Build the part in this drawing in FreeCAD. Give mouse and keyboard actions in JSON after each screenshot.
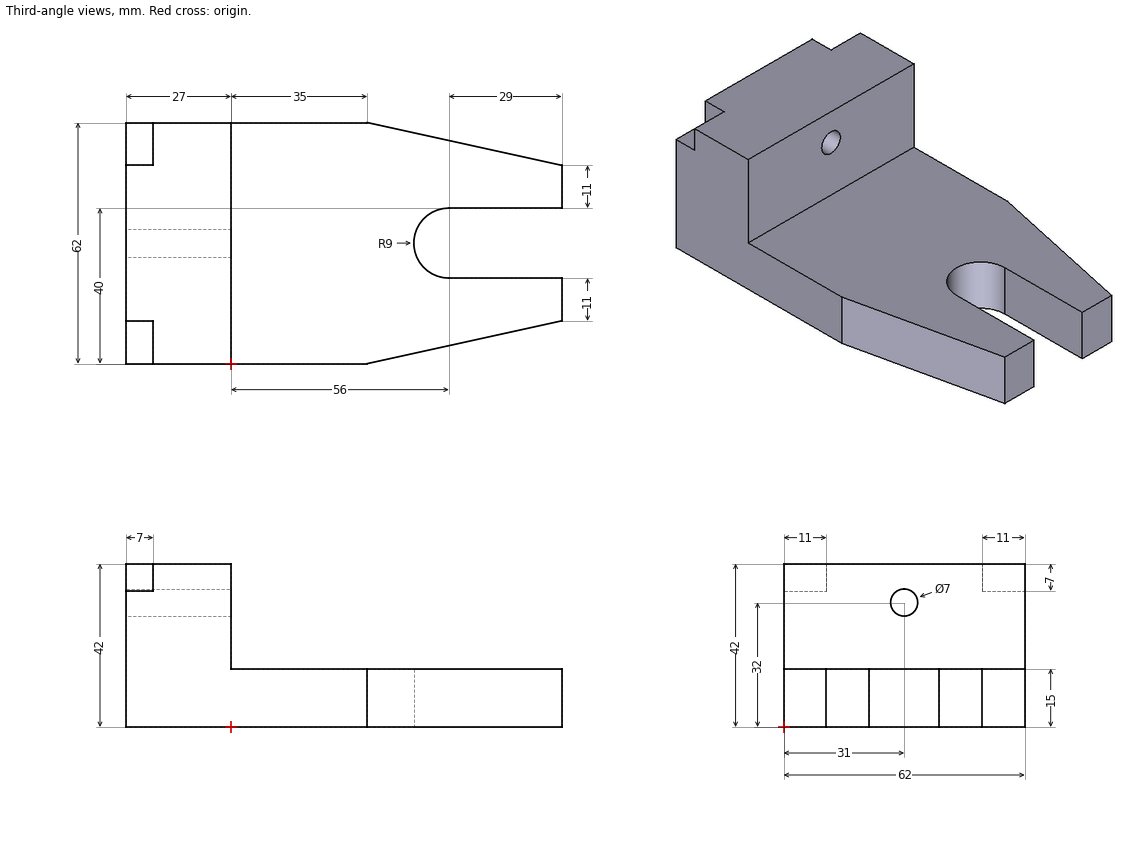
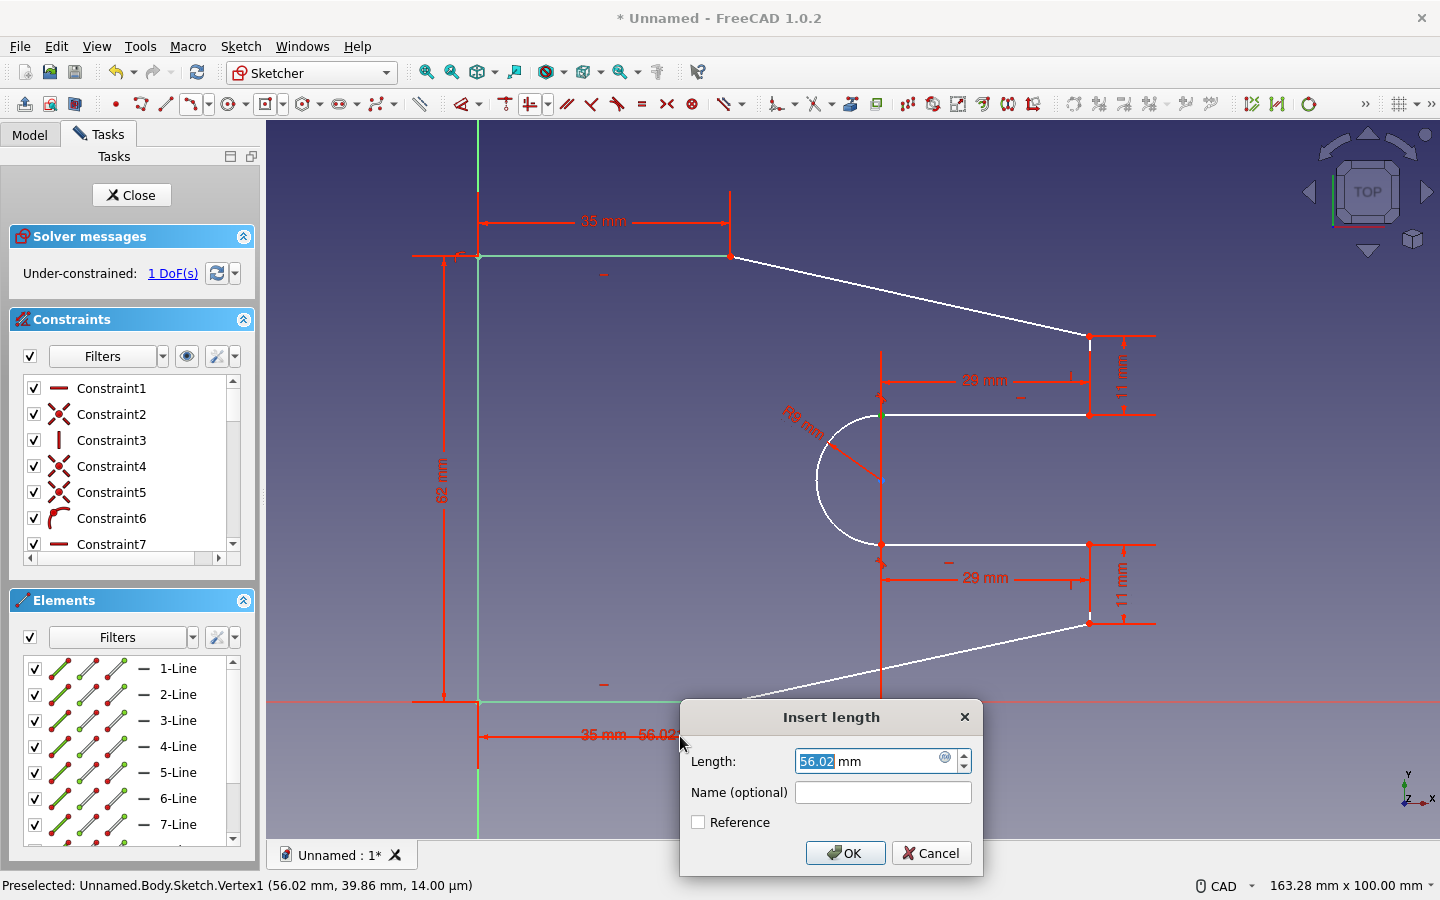
{"action": "type", "text": "56"}
{"action": "key", "text": "Return"}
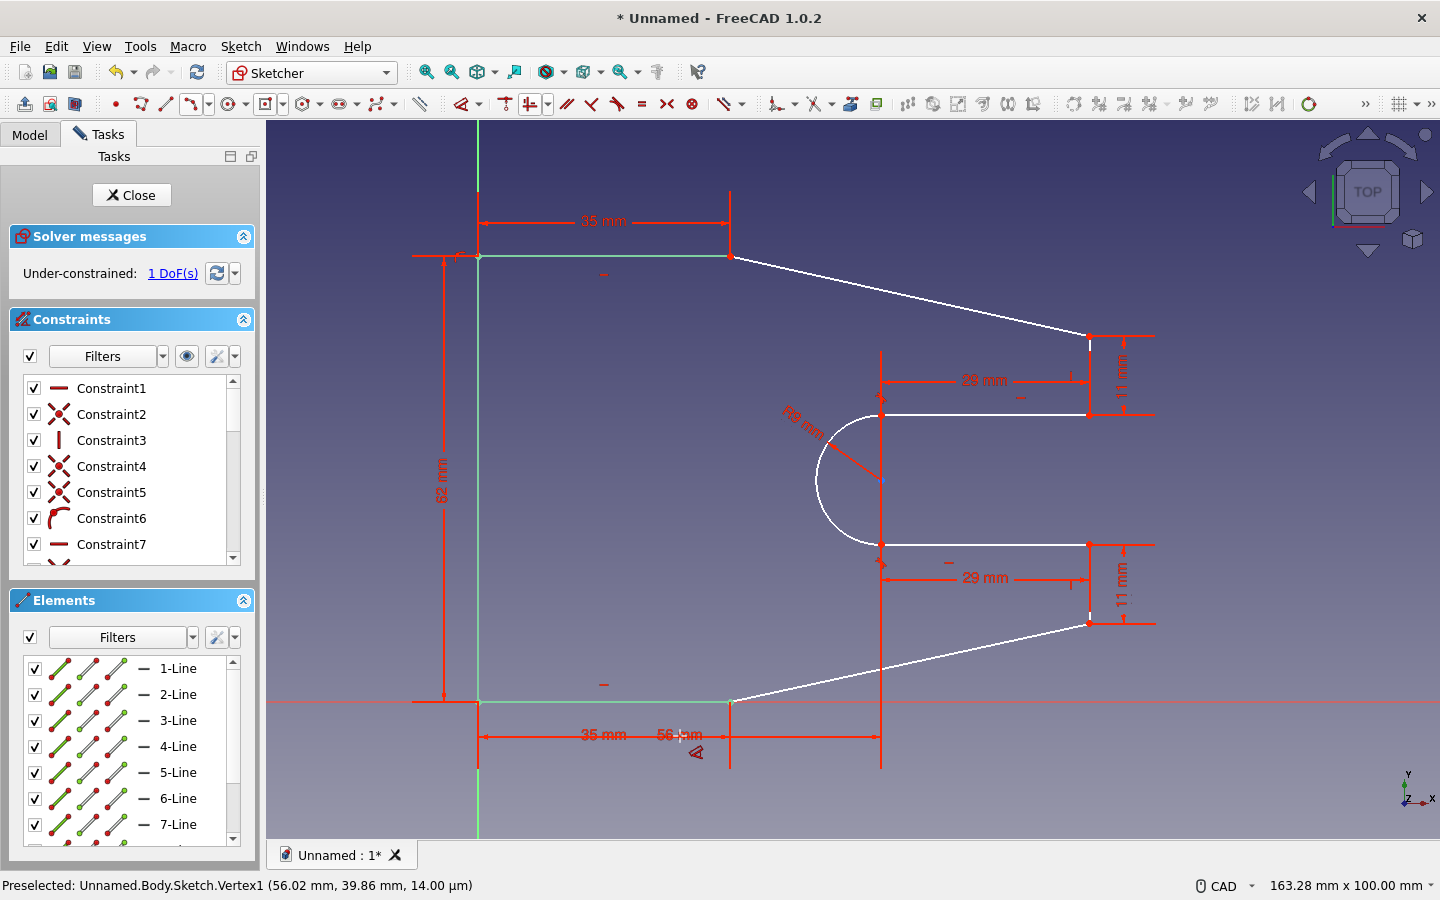
{"action": "left_click", "coordinate": [881, 415]}
{"action": "left_click", "coordinate": [444, 559]}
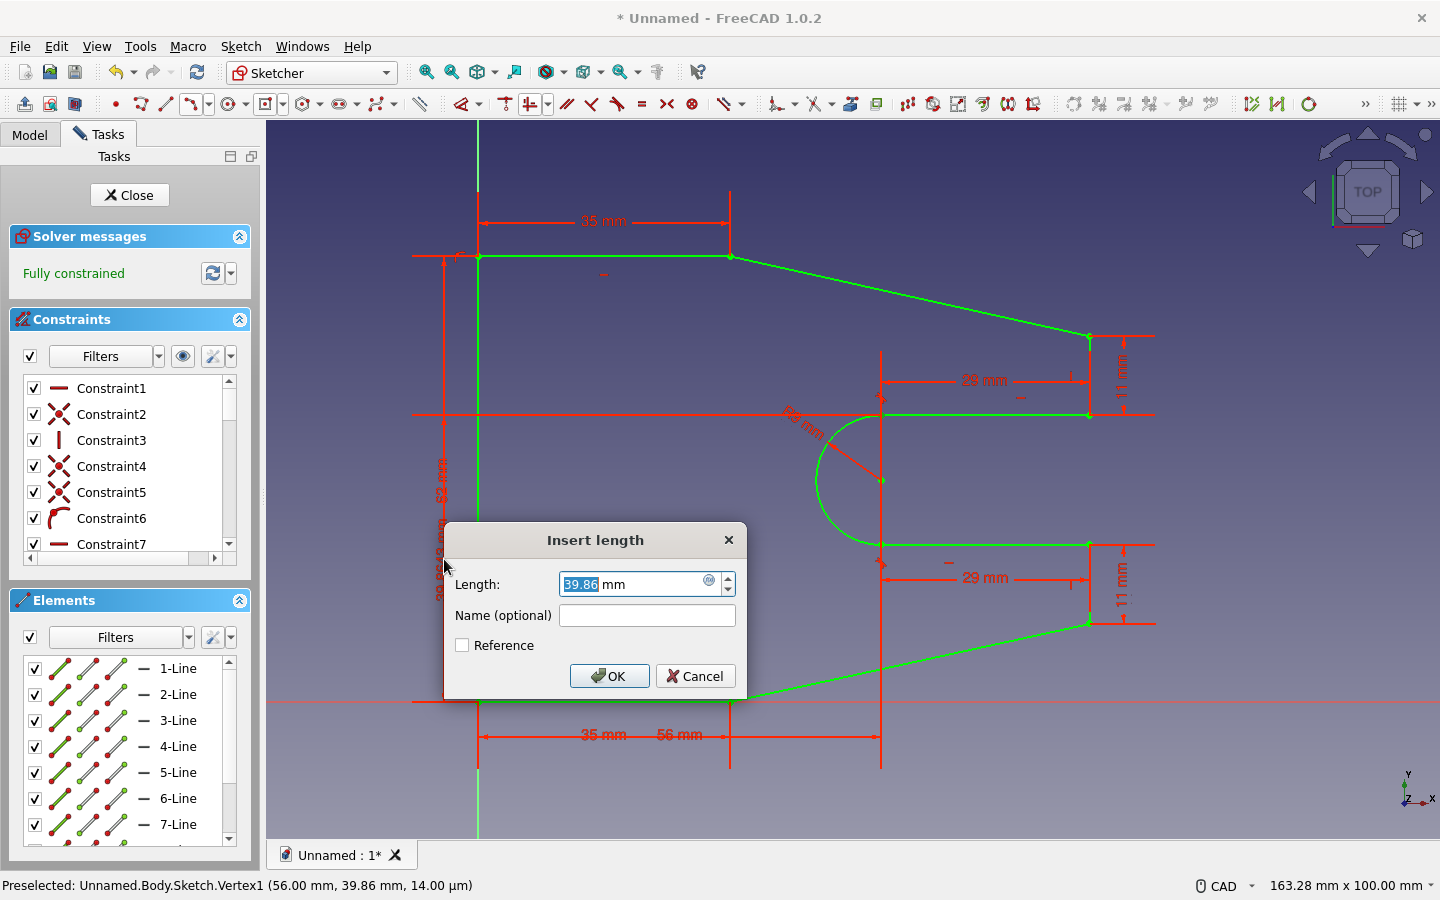
{"action": "type", "text": "40"}
{"action": "key", "text": "Return"}
{"action": "key", "text": "Escape"}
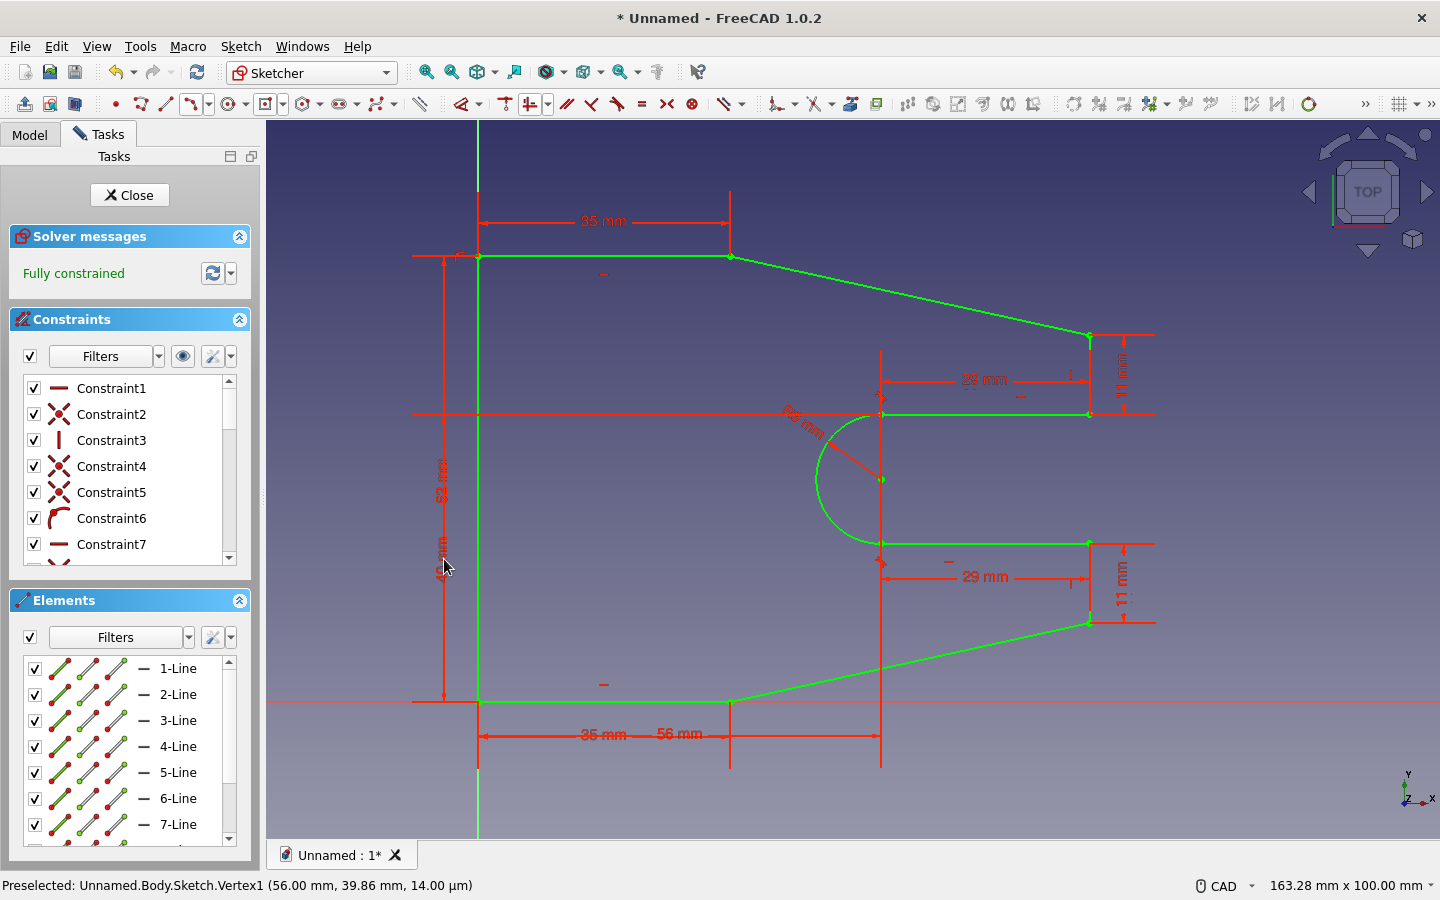
{"action": "left_click", "coordinate": [130, 195]}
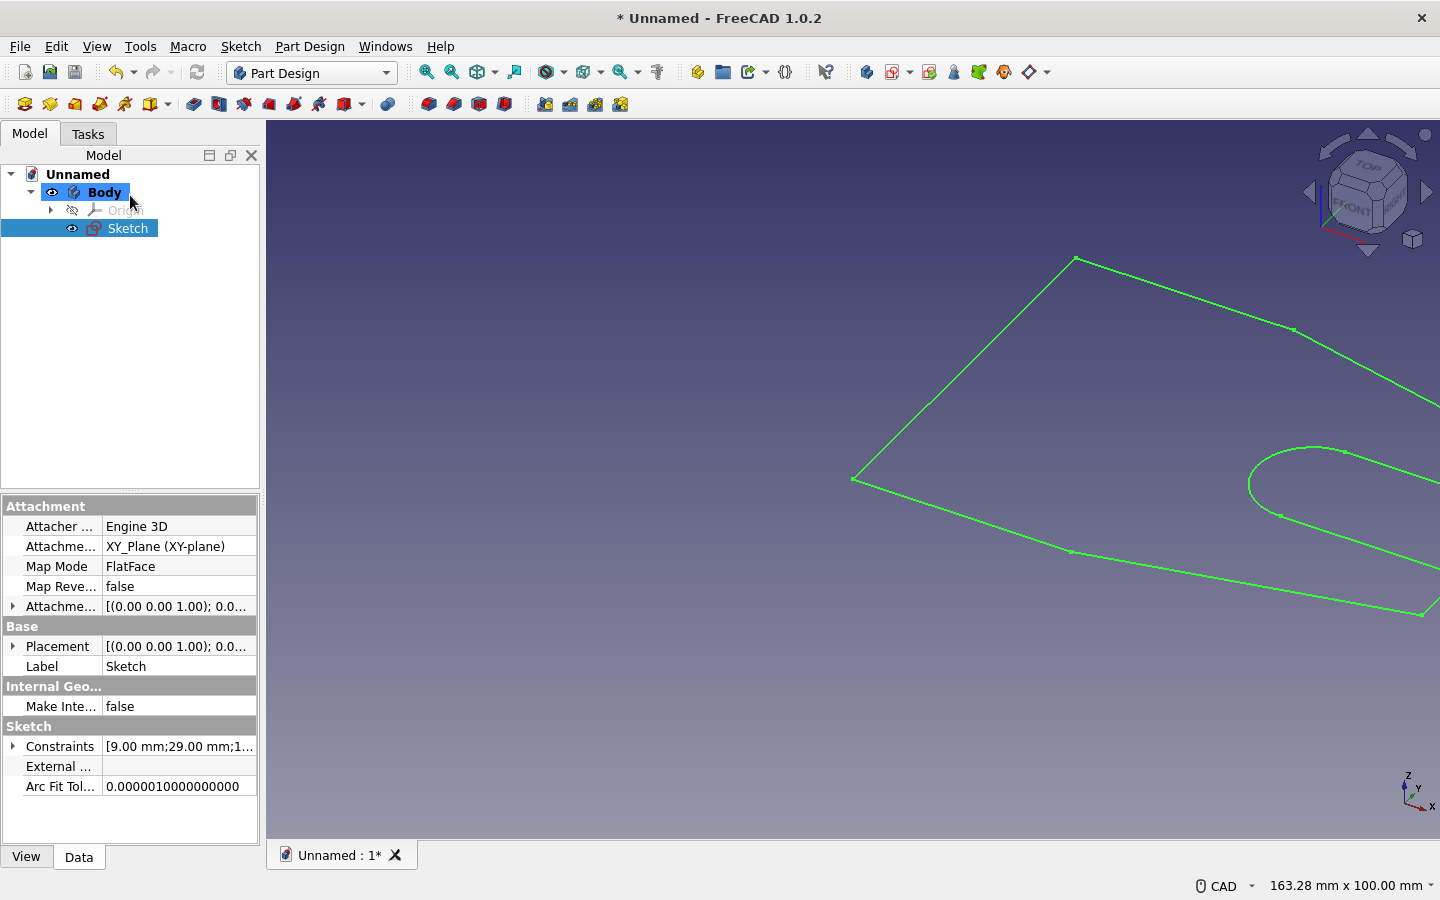
{"action": "left_click", "coordinate": [25, 104]}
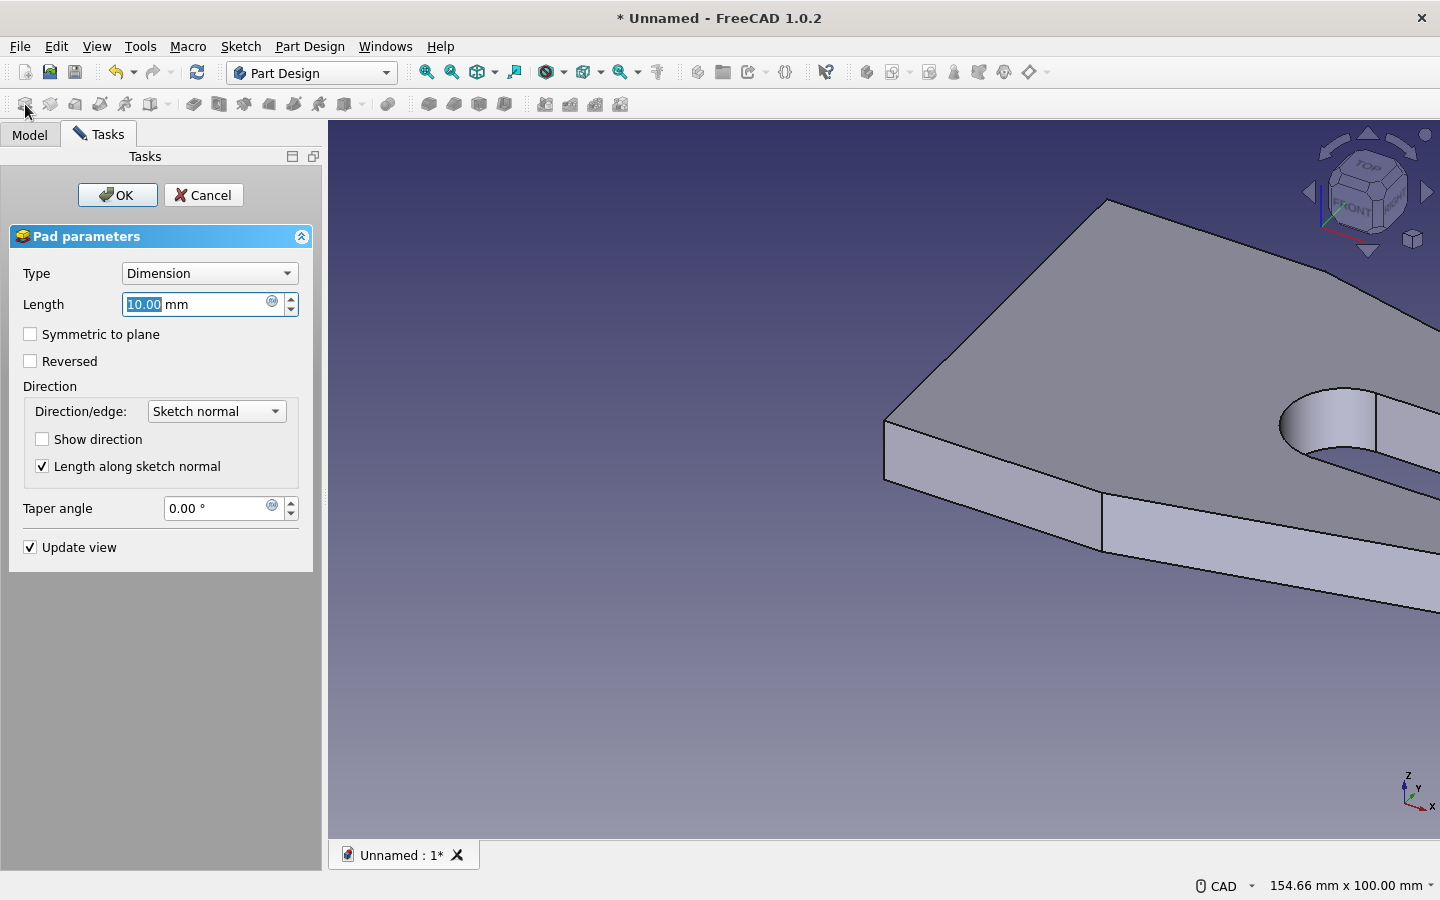
{"action": "type", "text": "15"}
{"action": "key", "text": "Tab"}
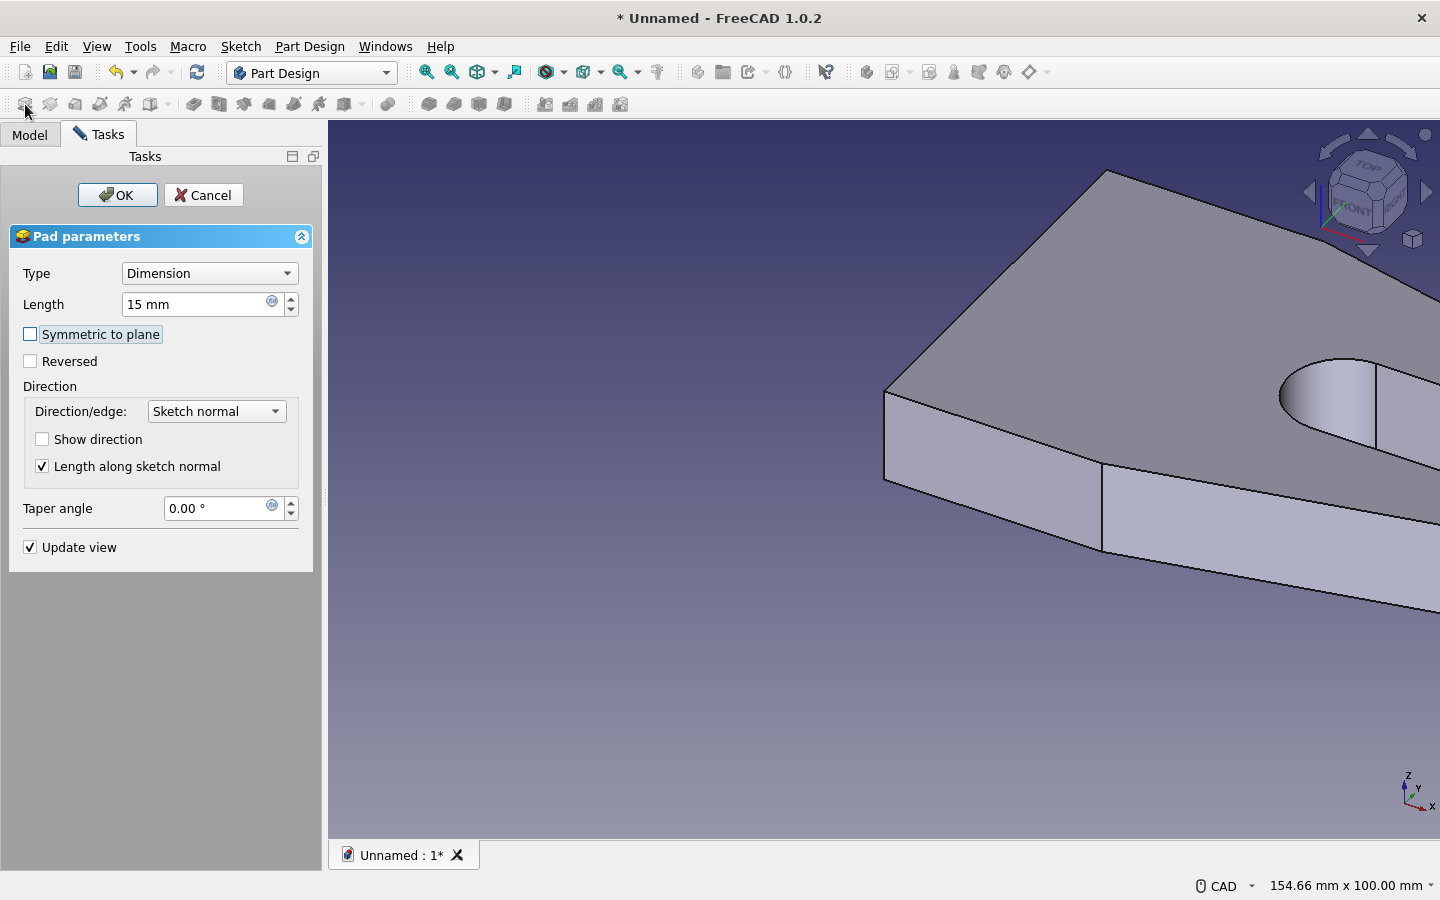
{"action": "left_click", "coordinate": [118, 195]}